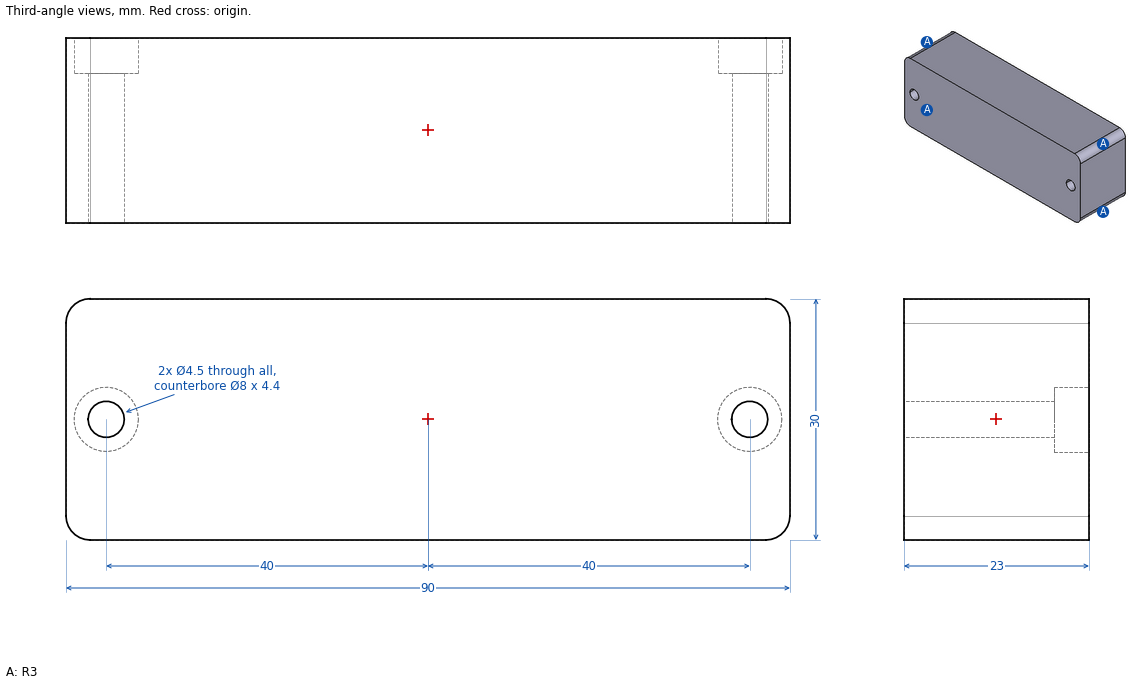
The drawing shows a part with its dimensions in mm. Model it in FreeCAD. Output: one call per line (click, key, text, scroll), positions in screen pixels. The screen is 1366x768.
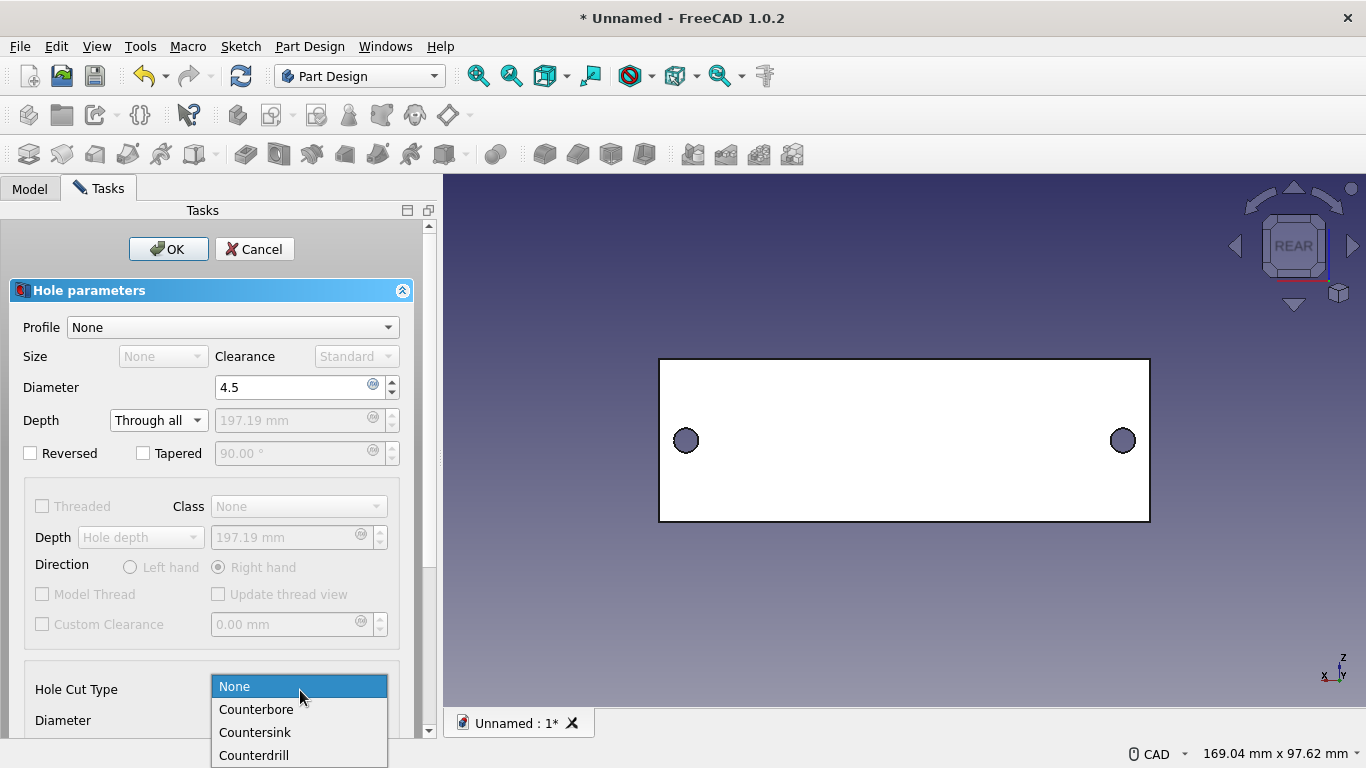
click(298, 710)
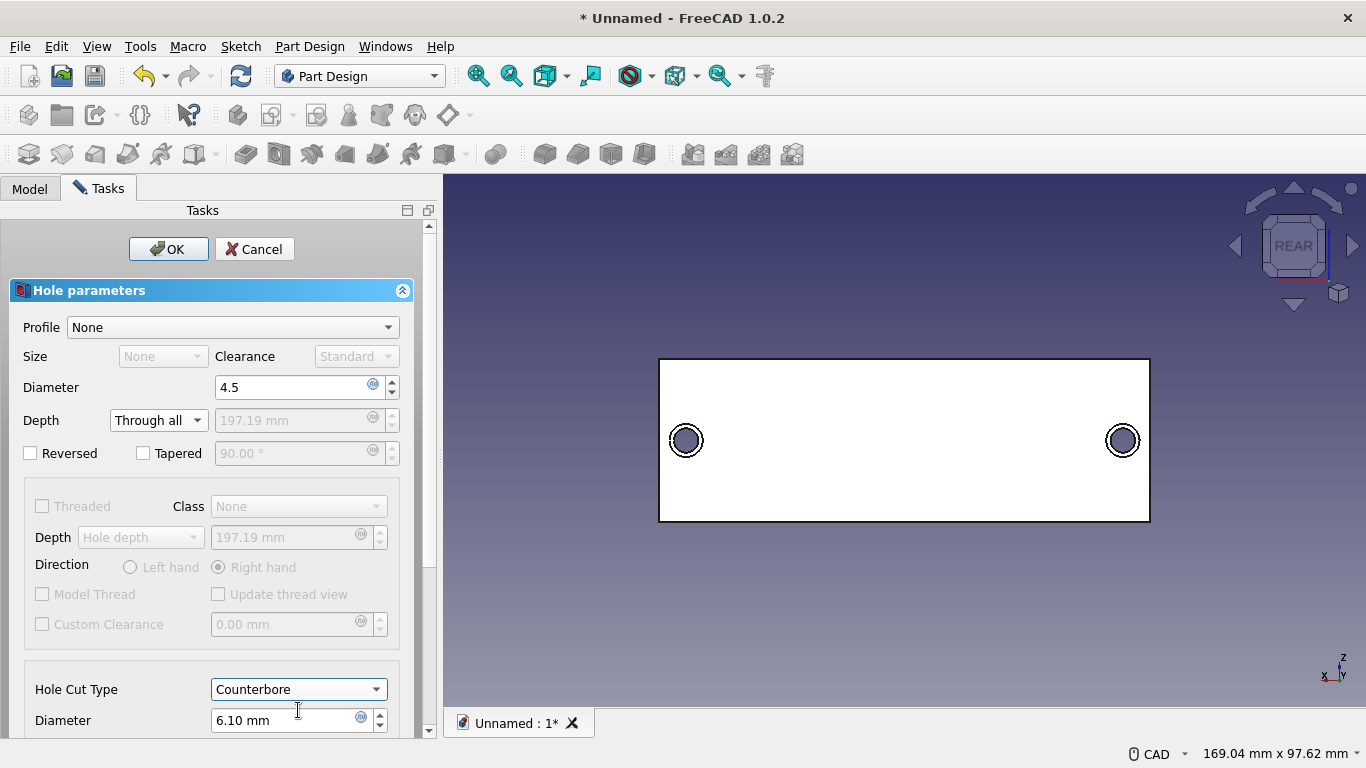
triple_click(292, 720)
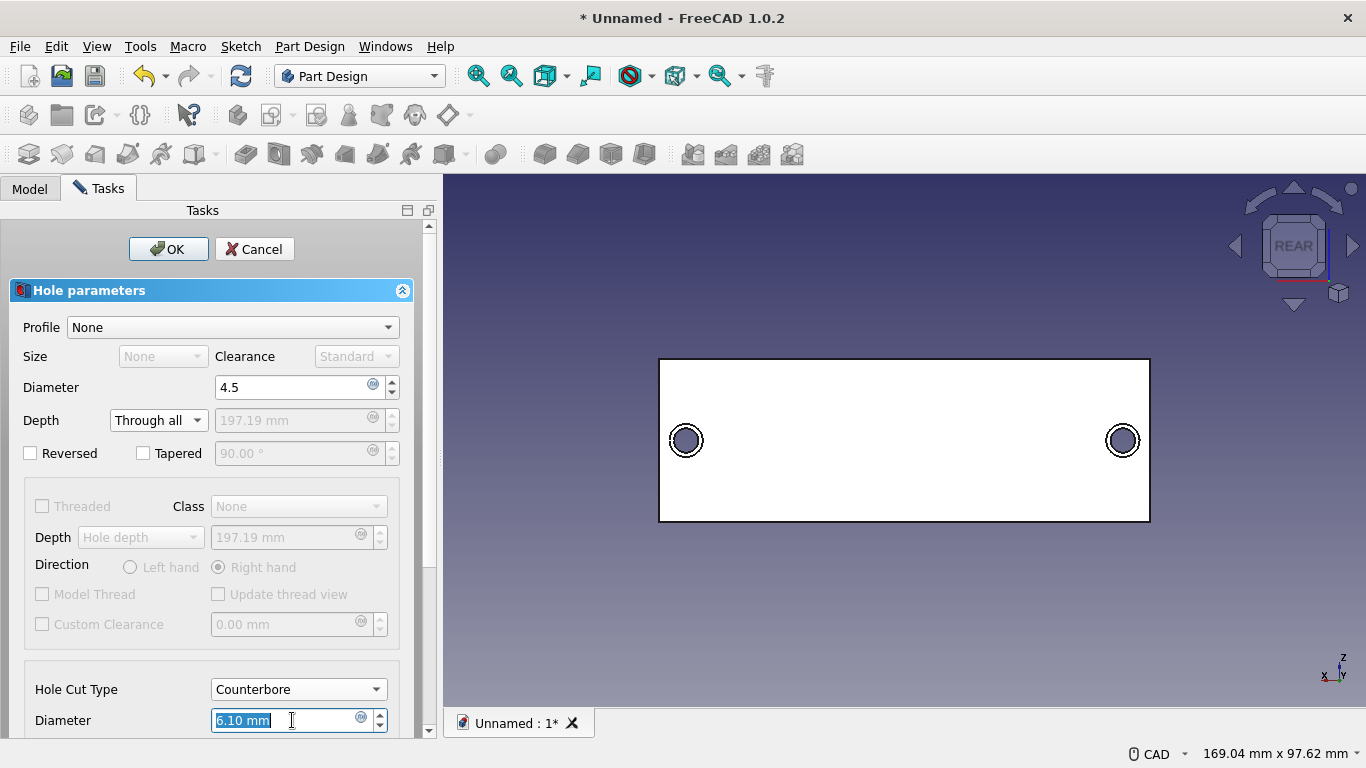
text(8)
key(Tab)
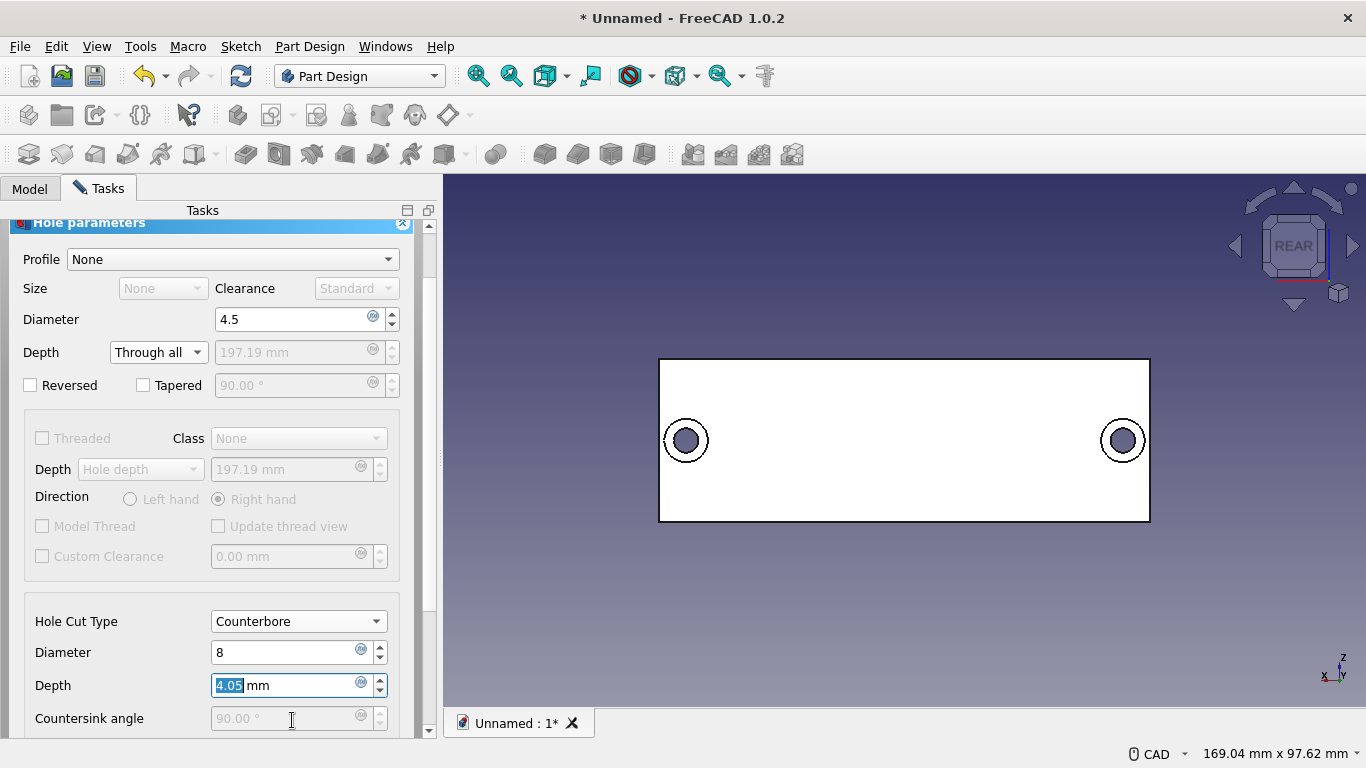
text(4.4)
key(Tab)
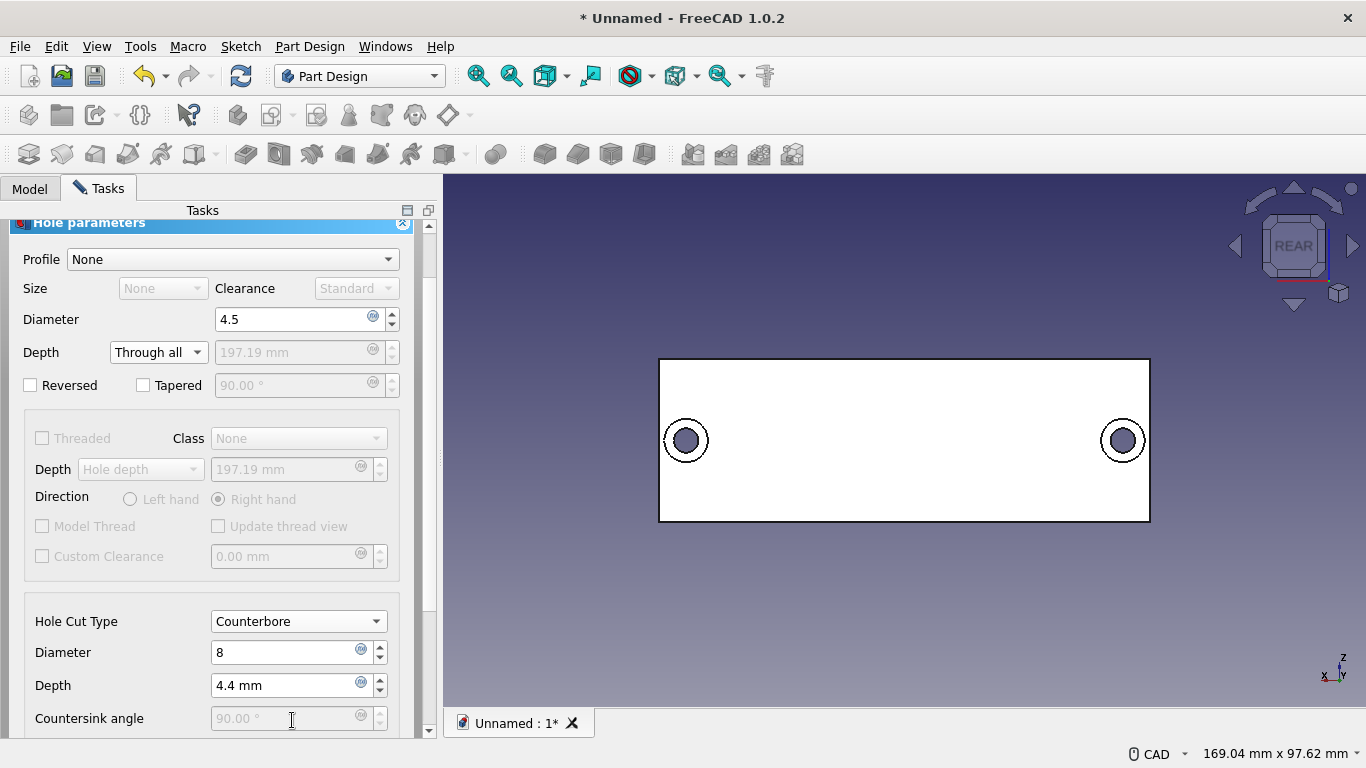
scroll(429, 479, up, 2)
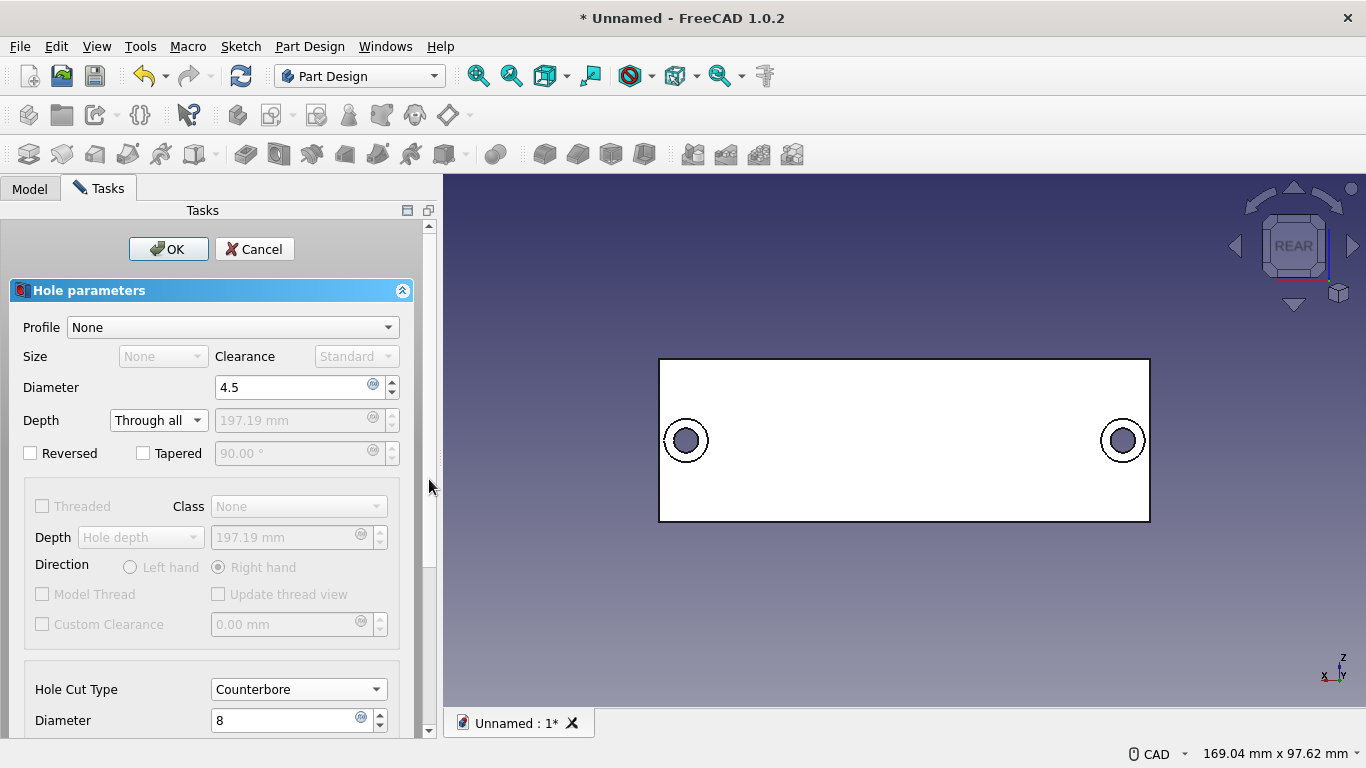
click(169, 249)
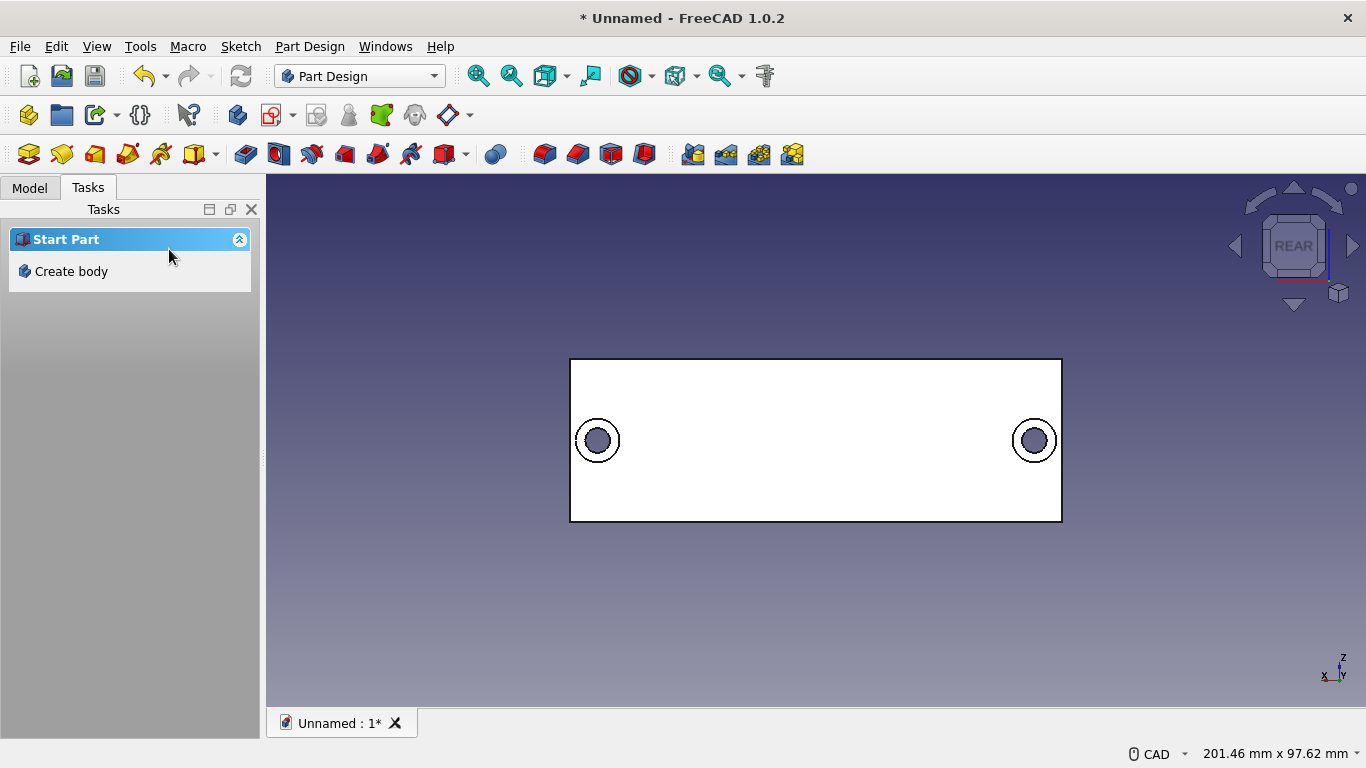
key(v)
key(f)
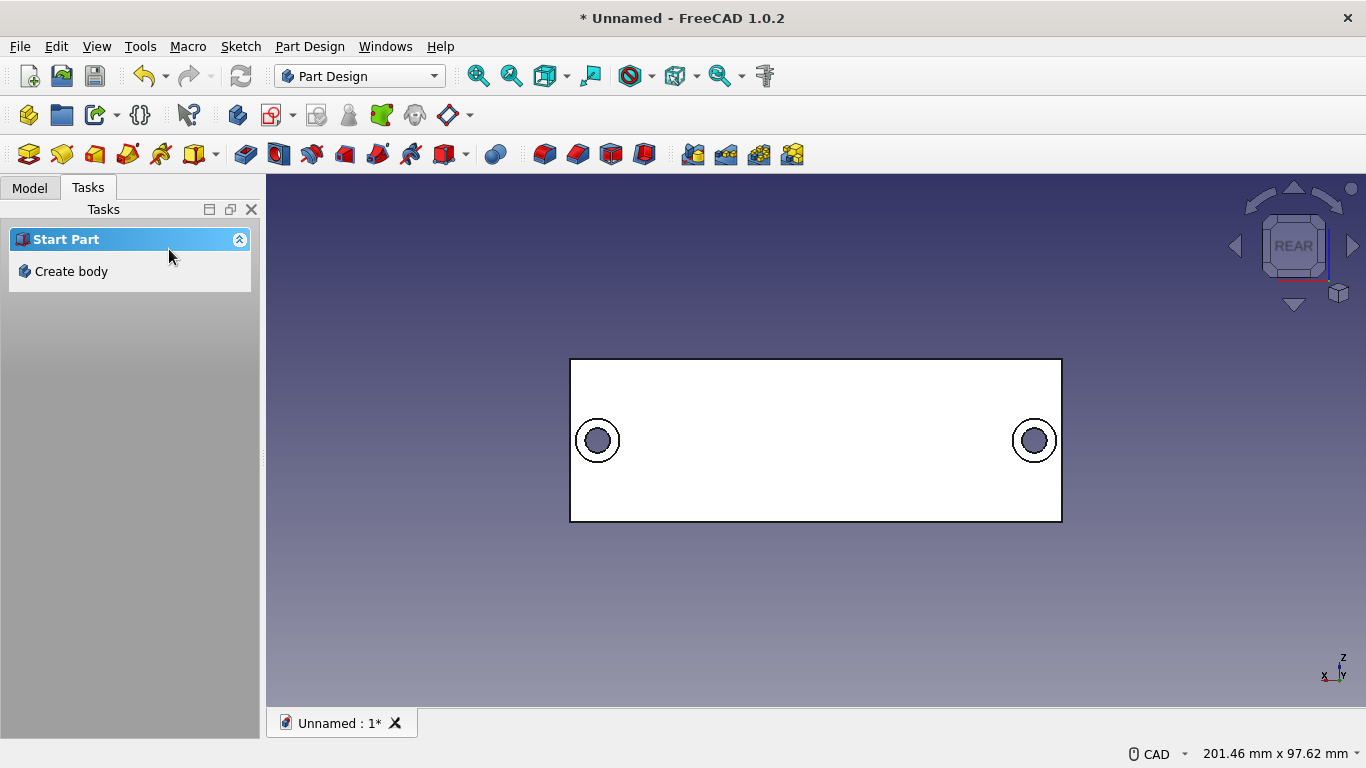
key(0)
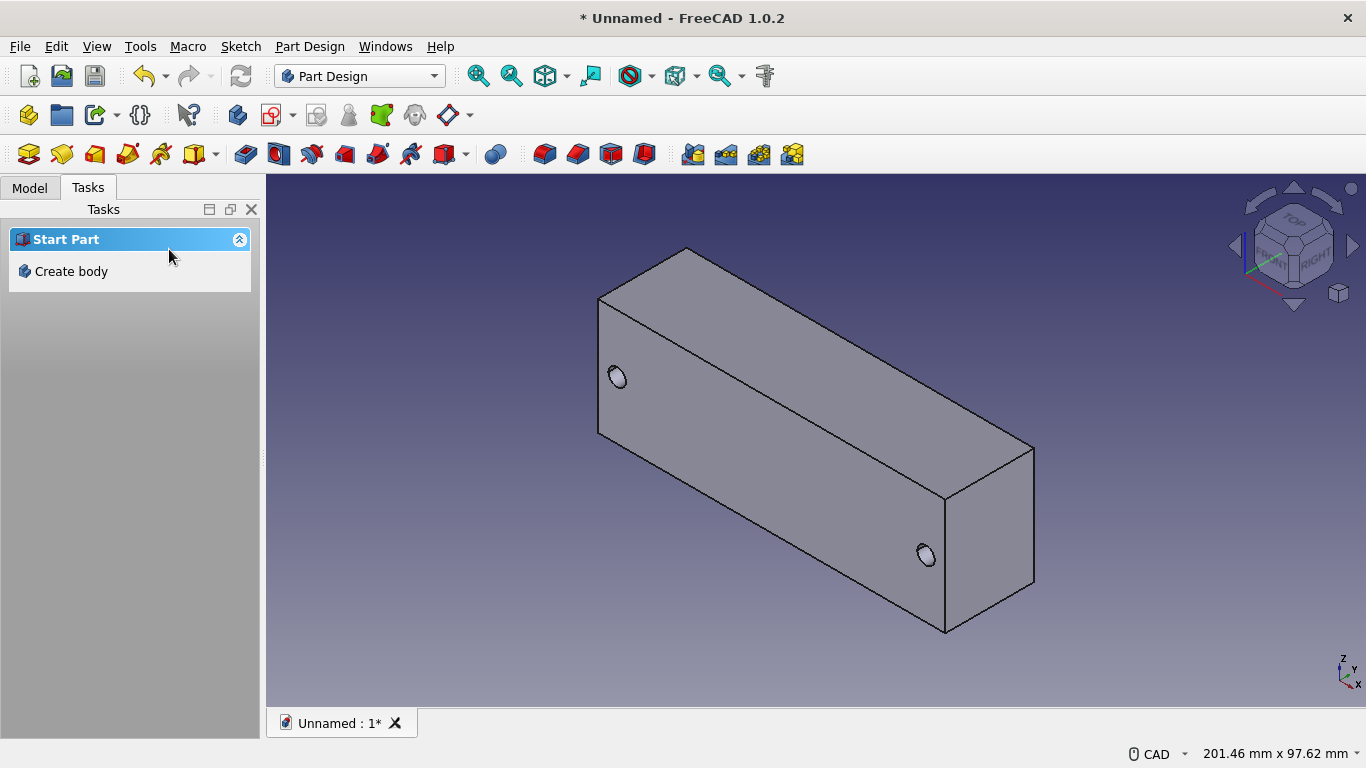
click(990, 473)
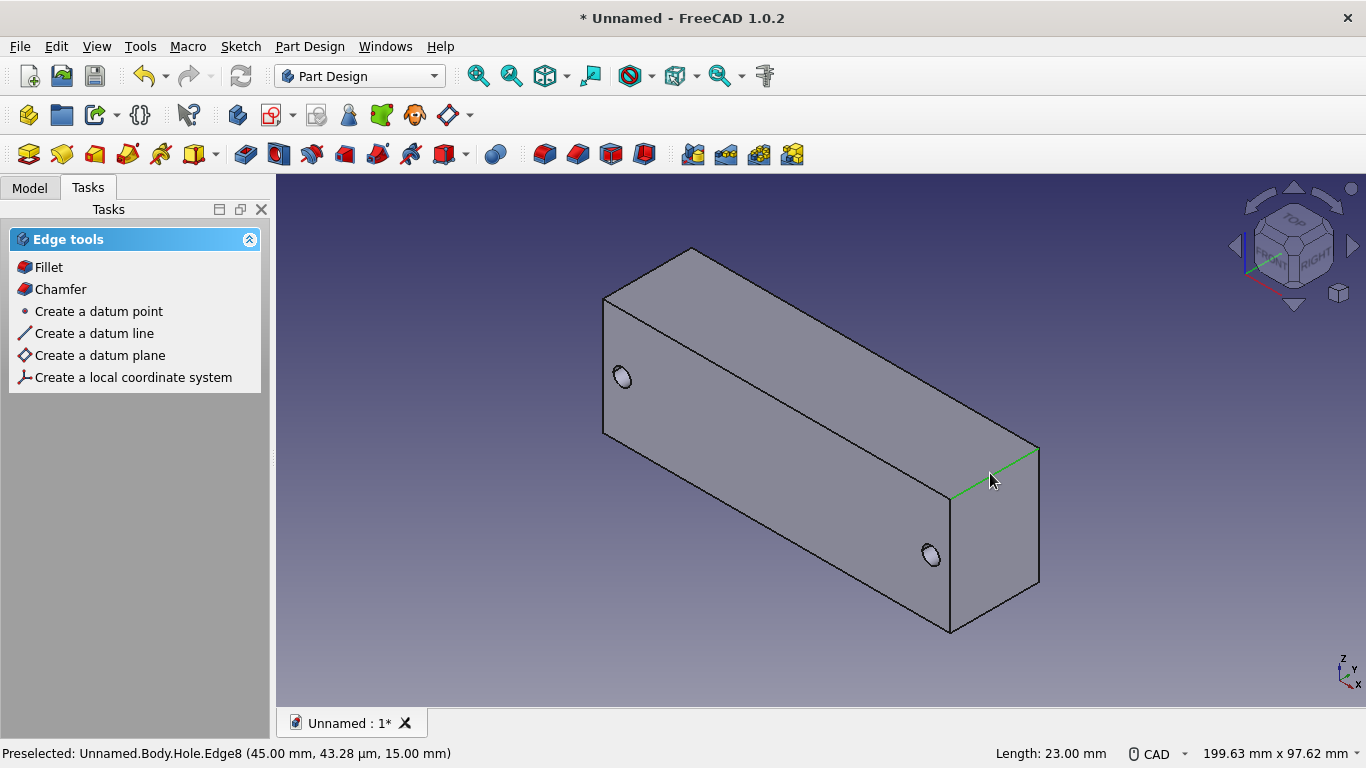
key(2)